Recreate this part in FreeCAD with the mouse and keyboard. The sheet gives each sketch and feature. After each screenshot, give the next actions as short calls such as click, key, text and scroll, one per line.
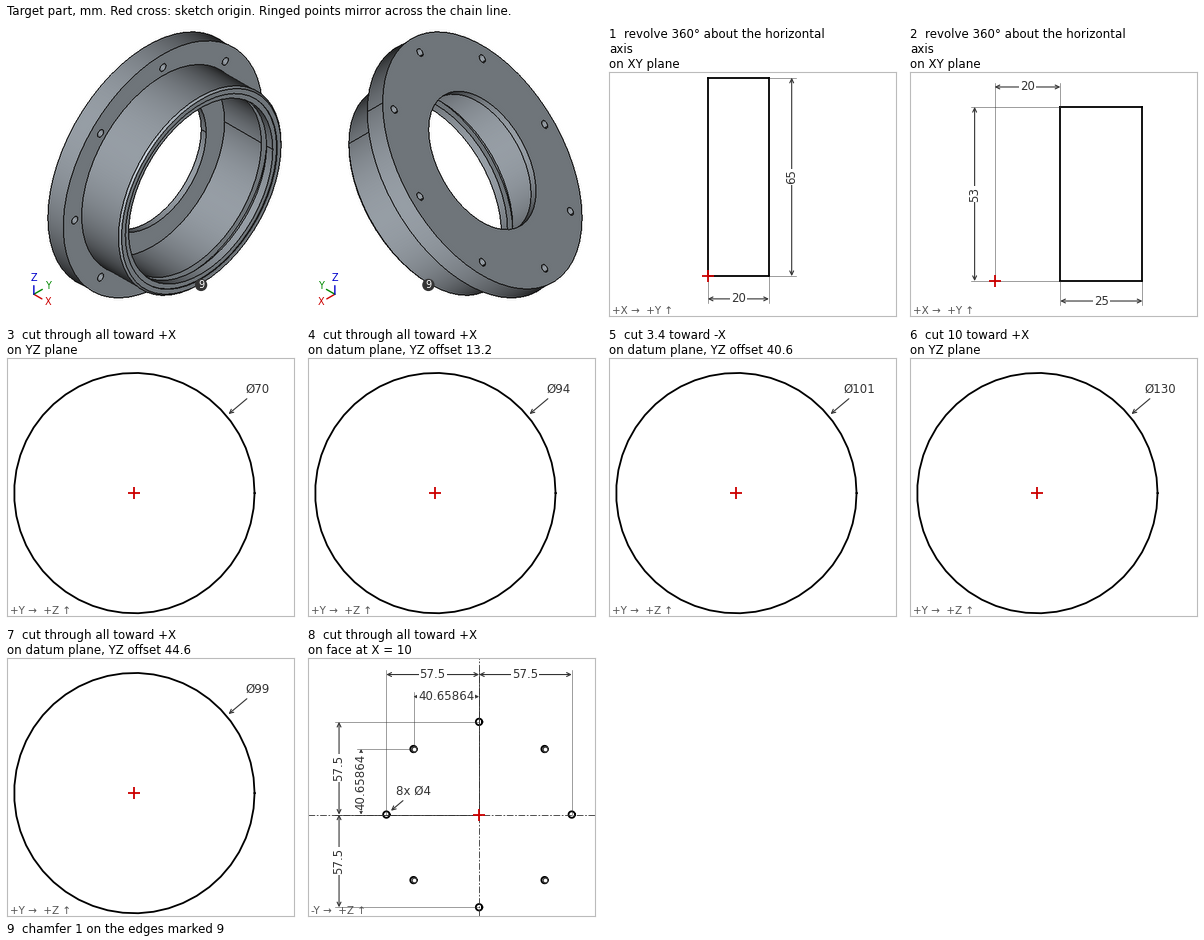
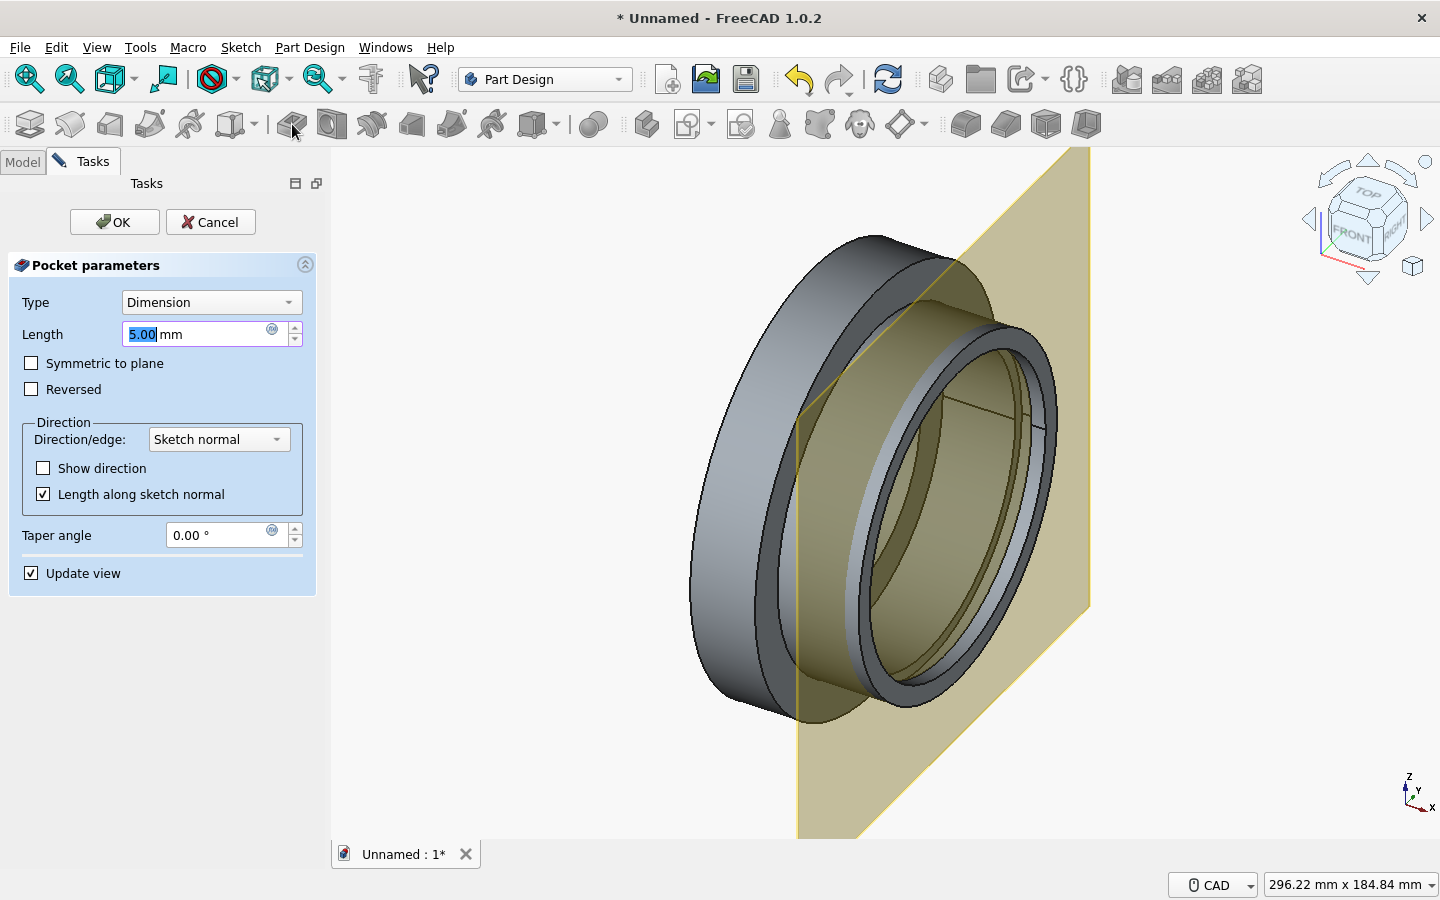
text(3.4)
key(Tab)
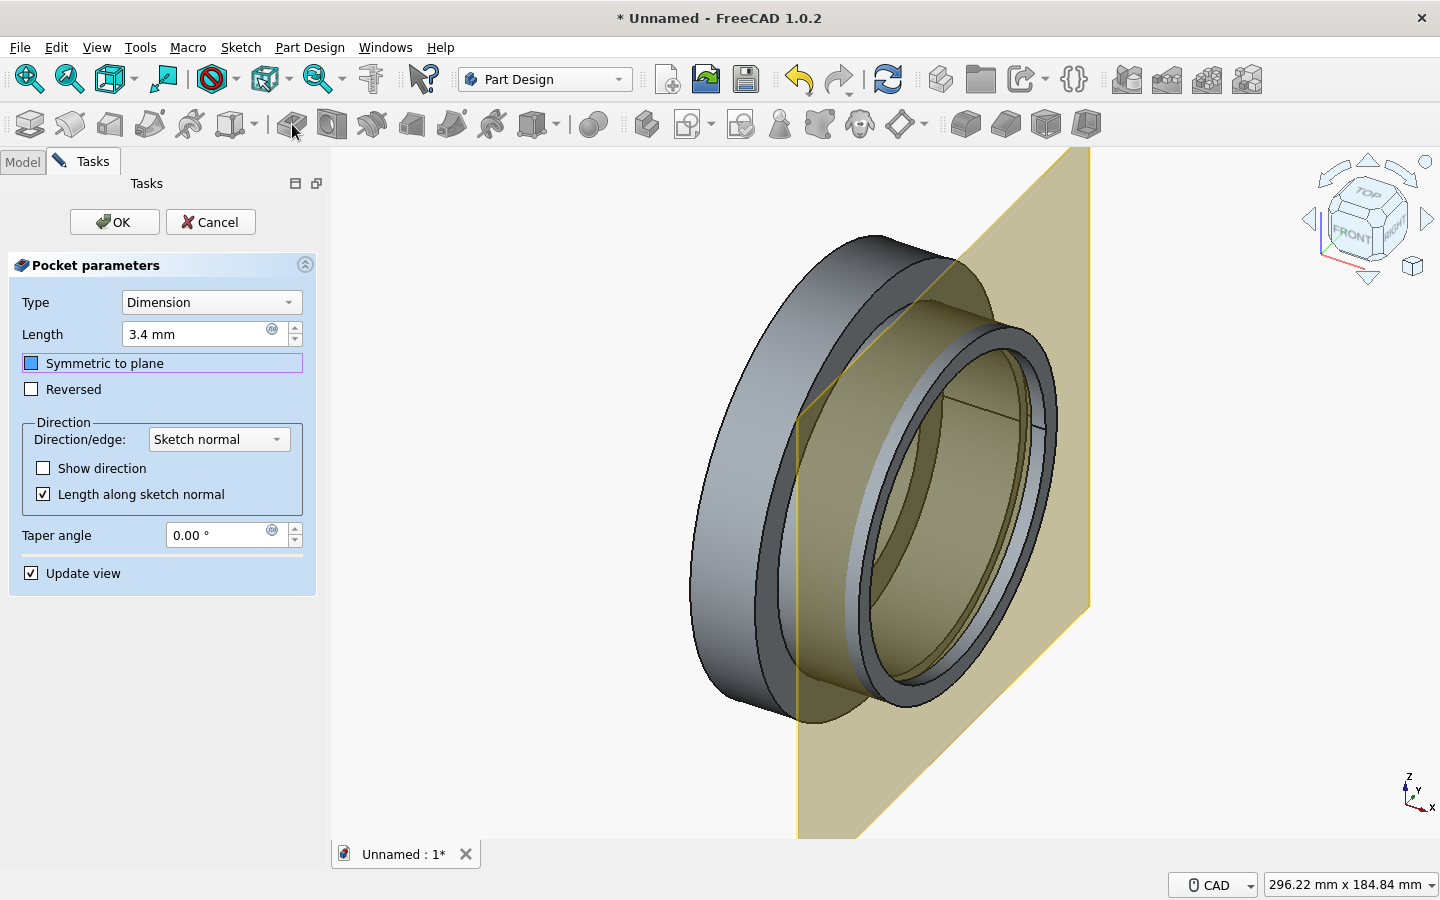
click(115, 222)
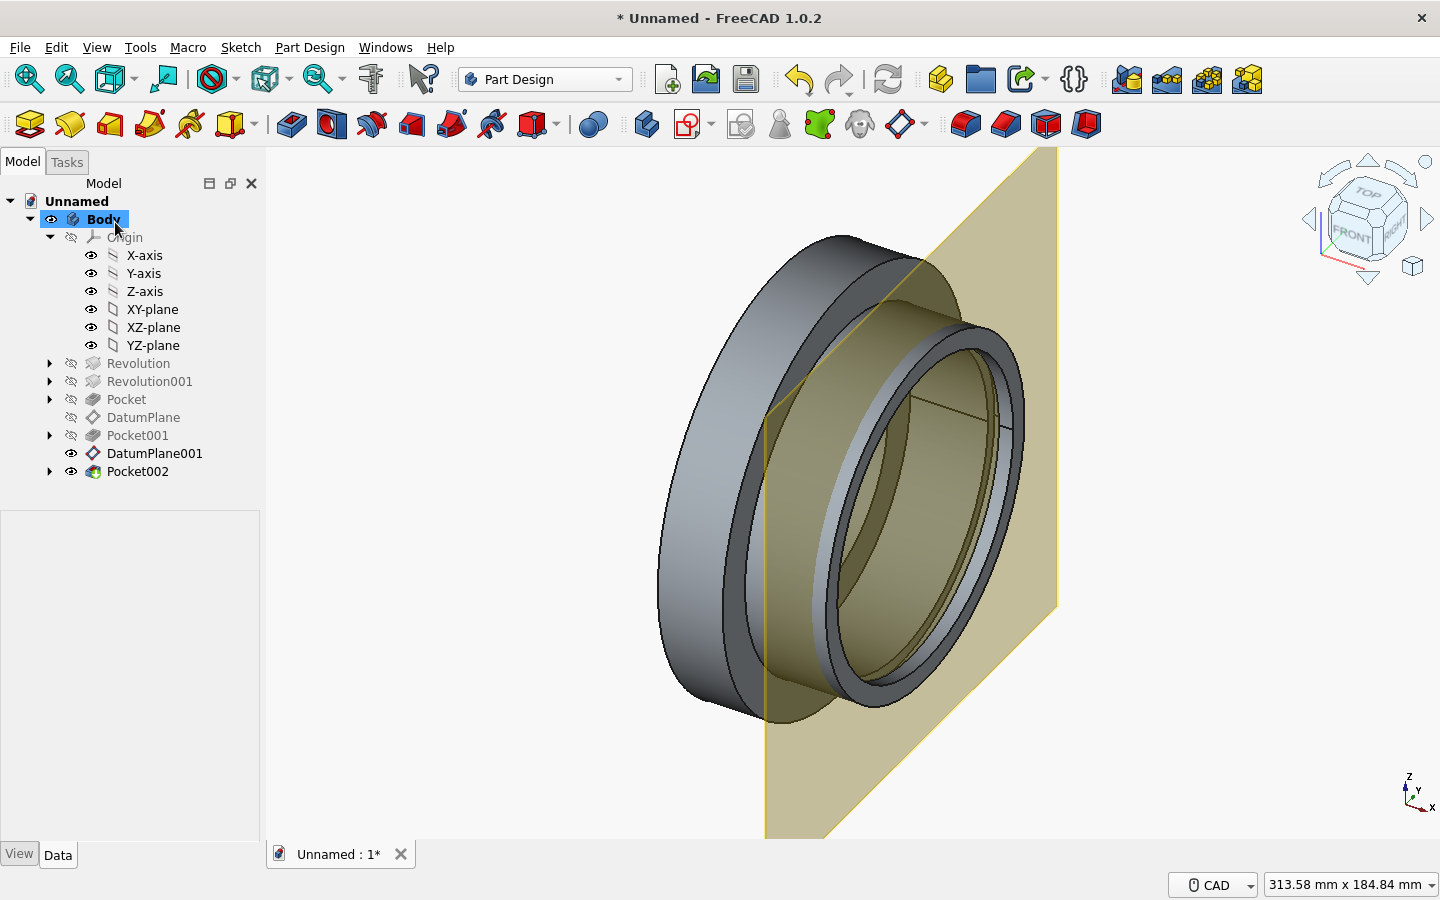
click(116, 453)
key(space)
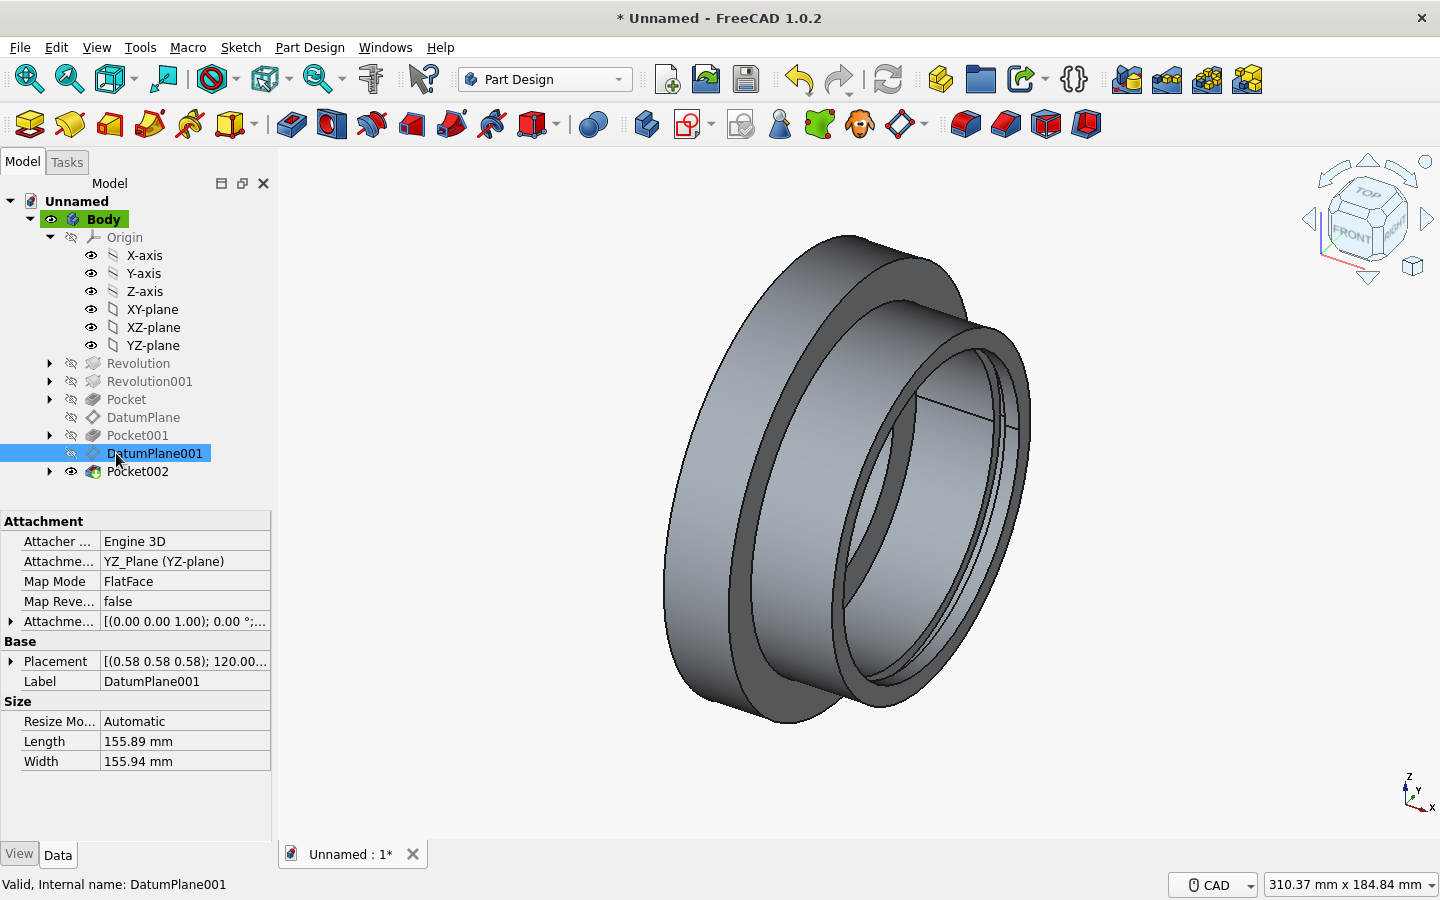
click(318, 799)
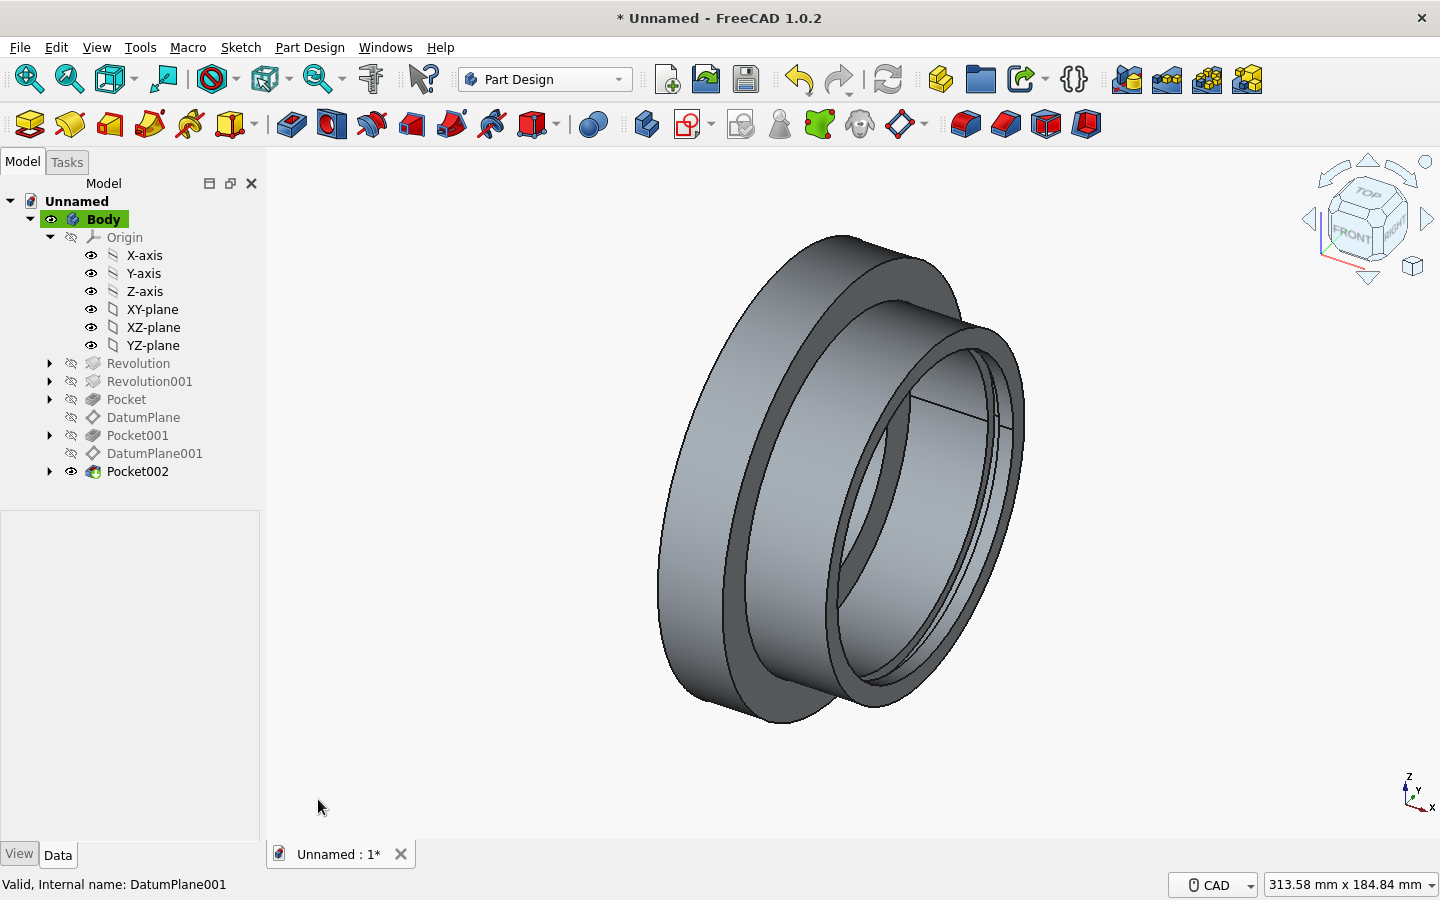
click(688, 124)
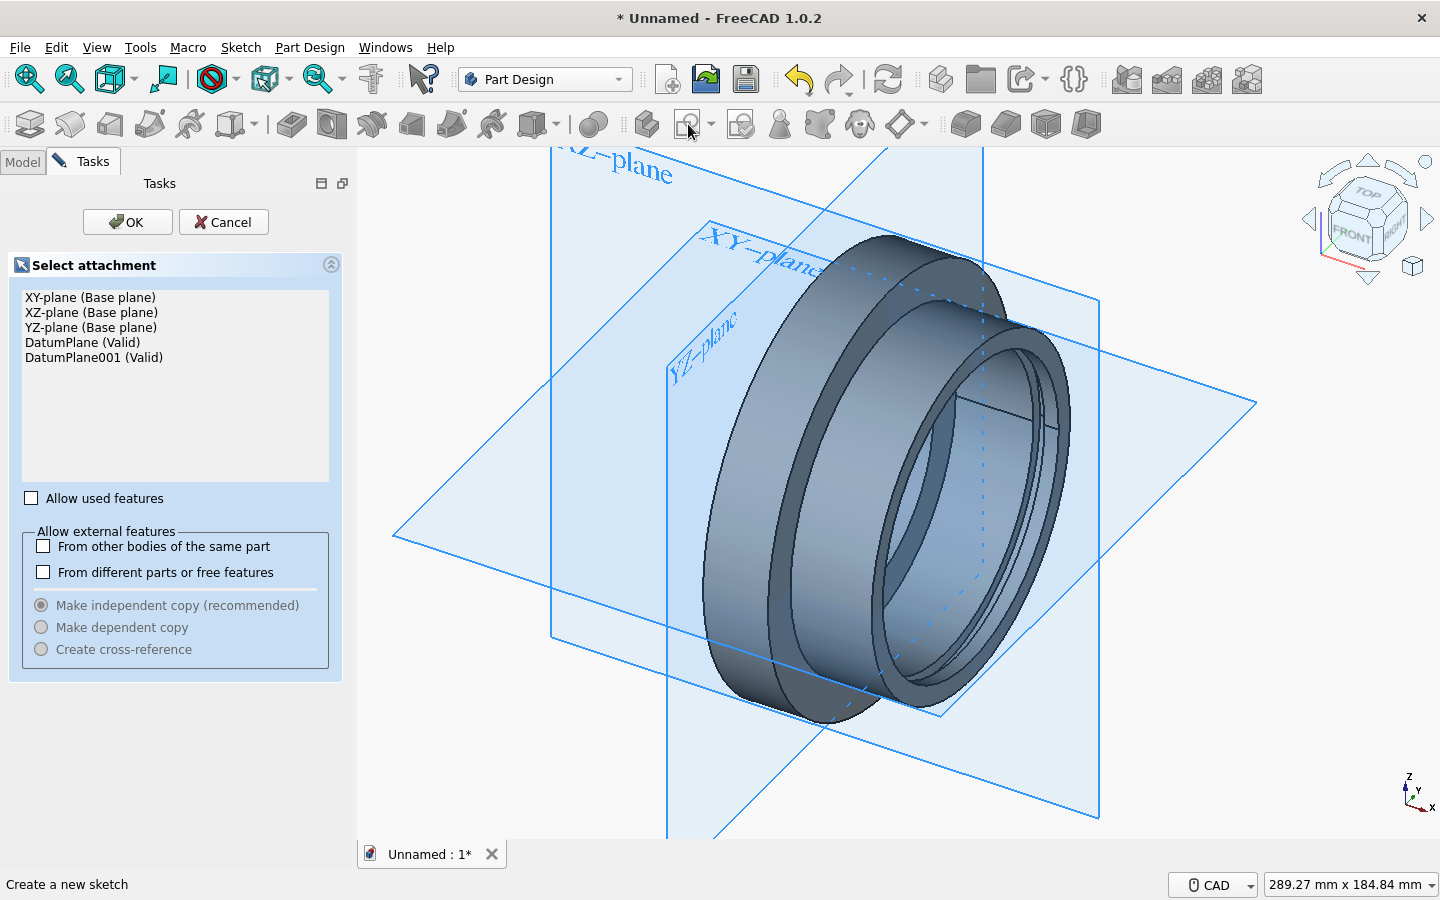
click(82, 328)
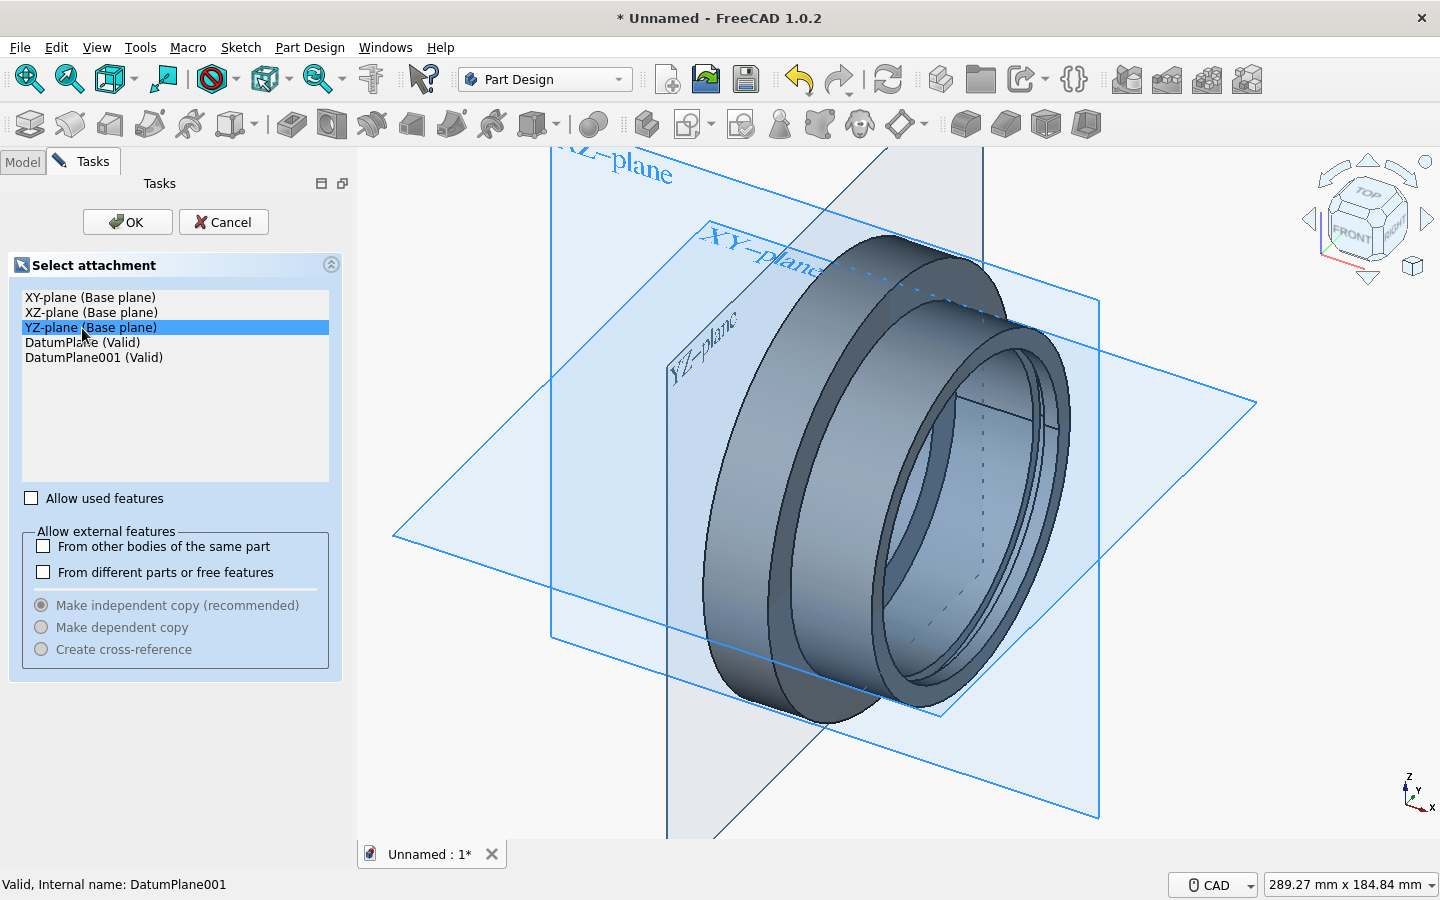
click(128, 222)